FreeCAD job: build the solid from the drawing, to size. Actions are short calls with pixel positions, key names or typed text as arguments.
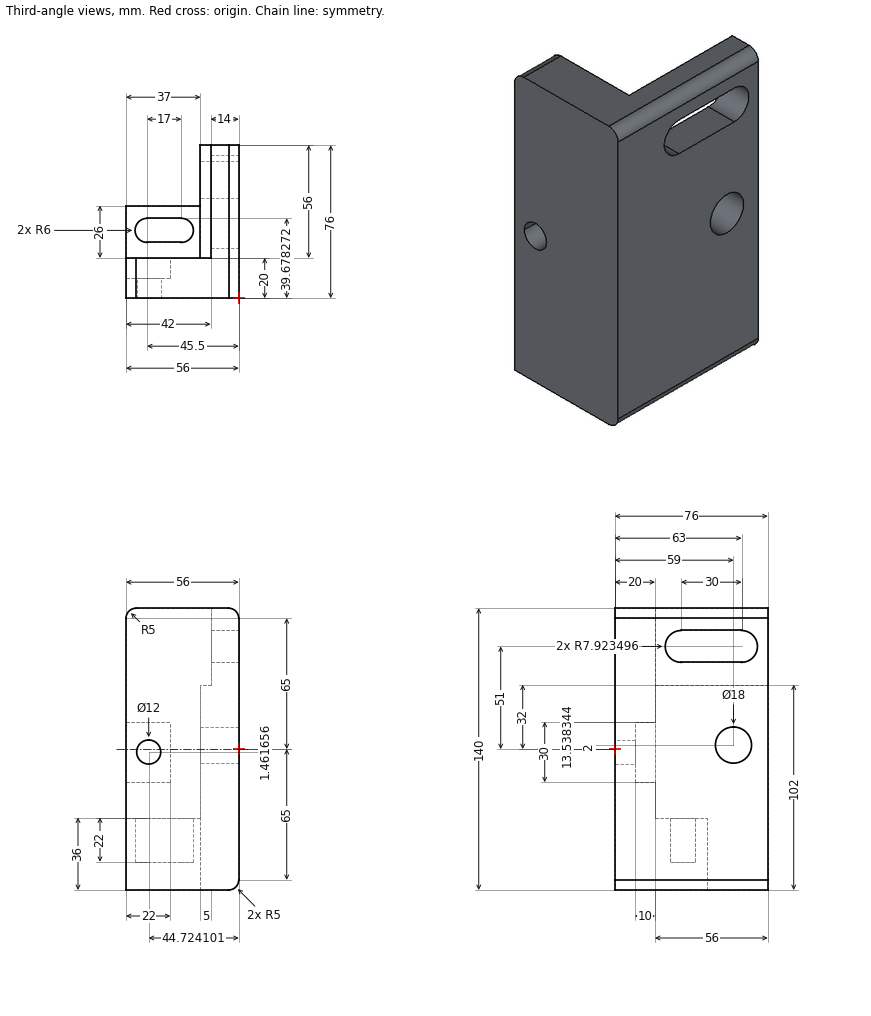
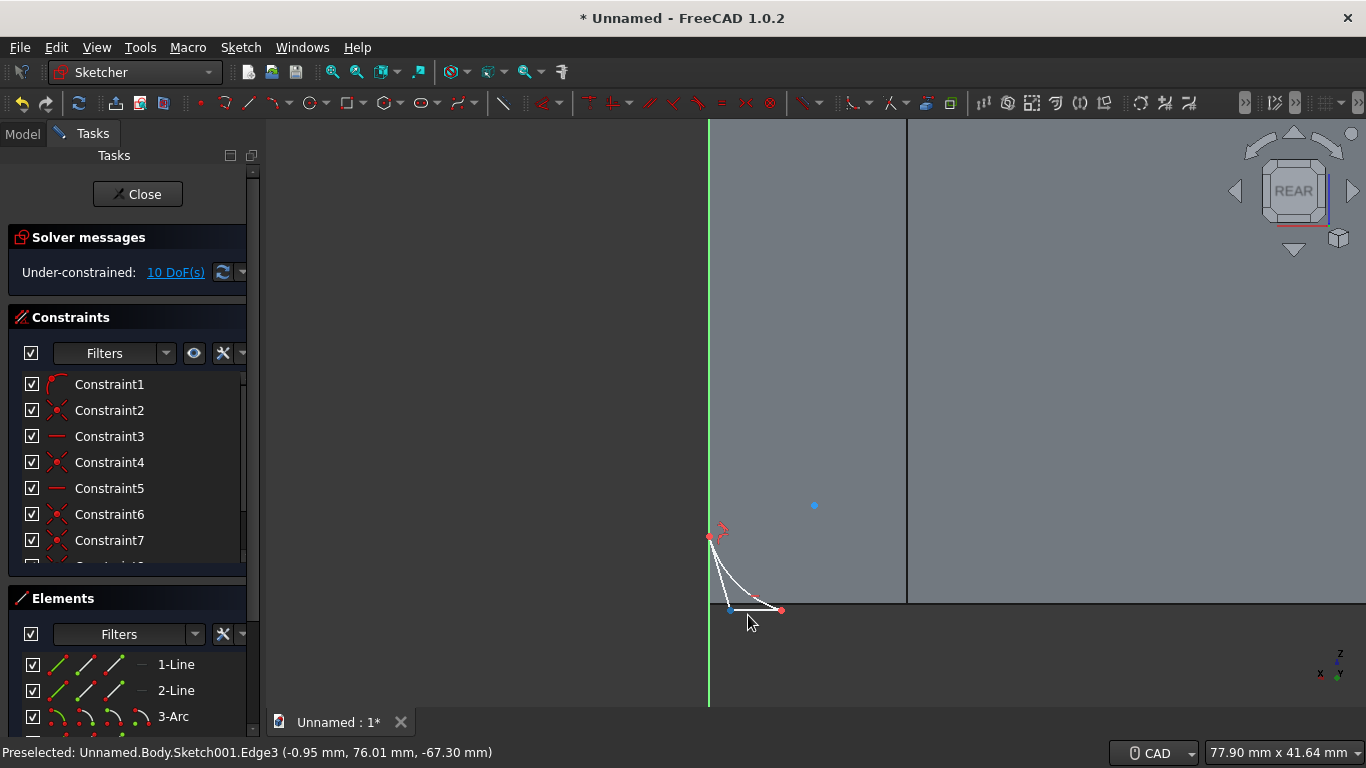
click(746, 610)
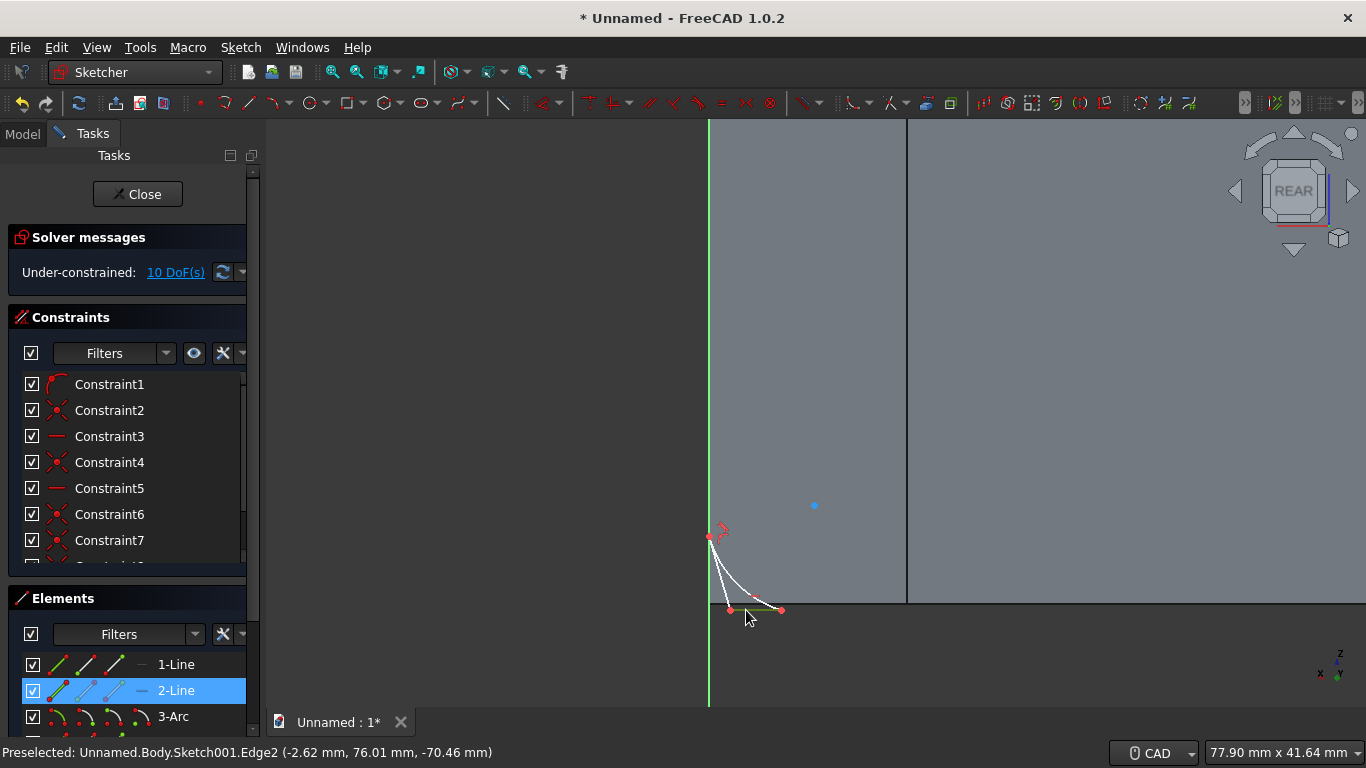
click(736, 582)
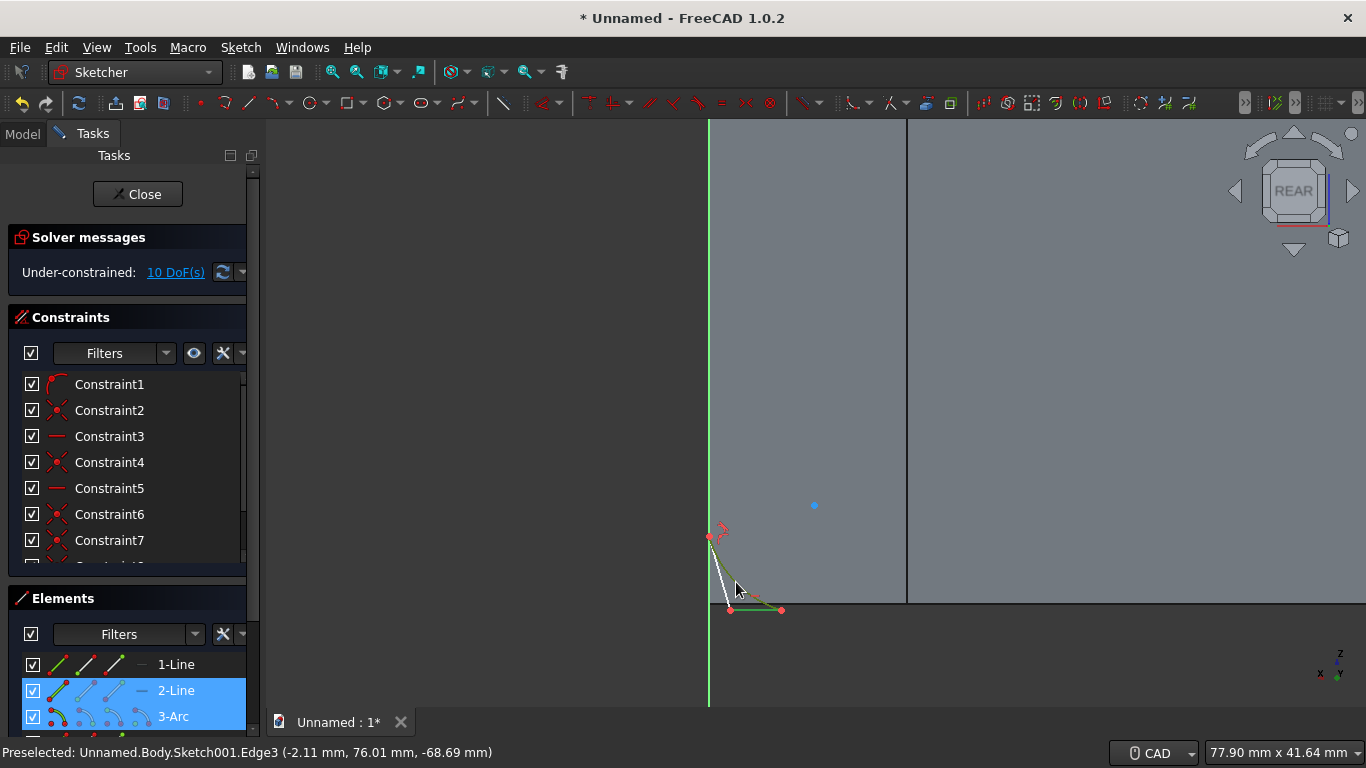
click(698, 104)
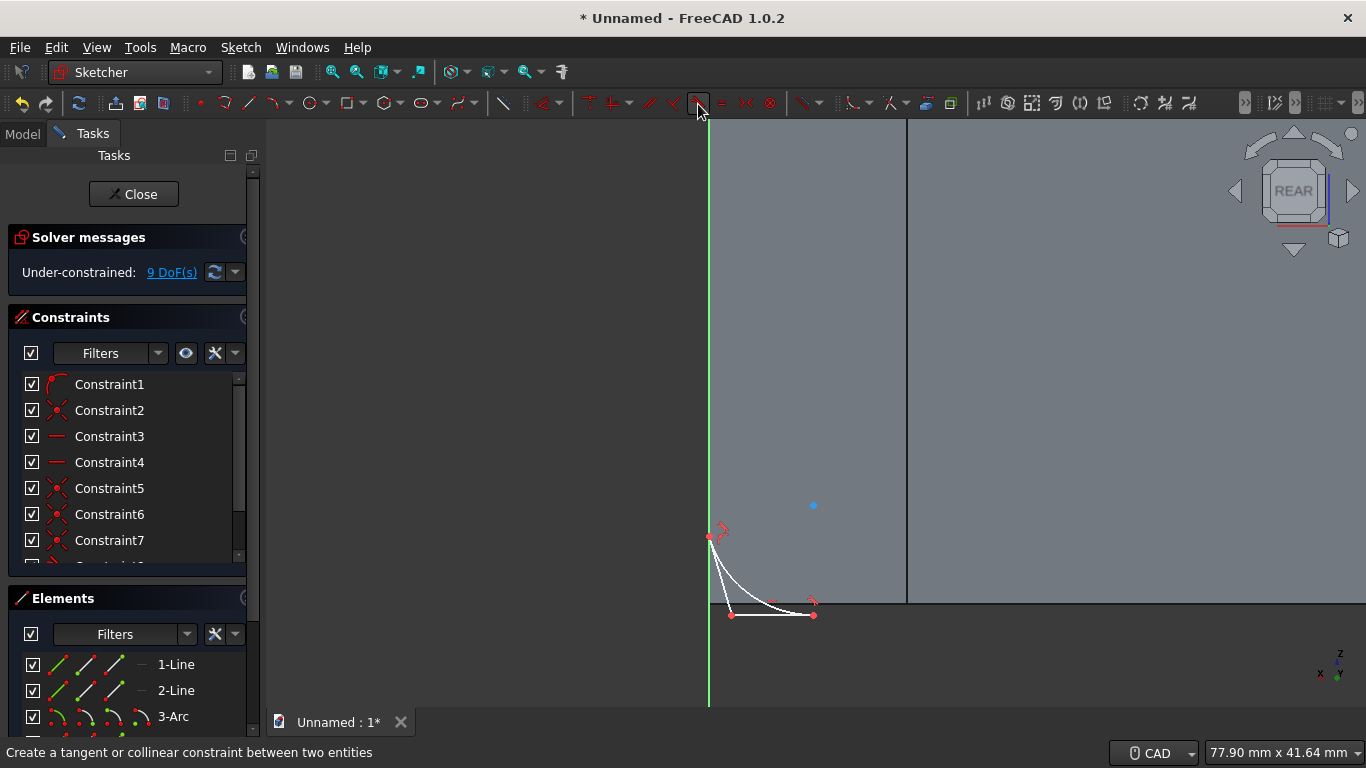
scroll(748, 615, down, 8)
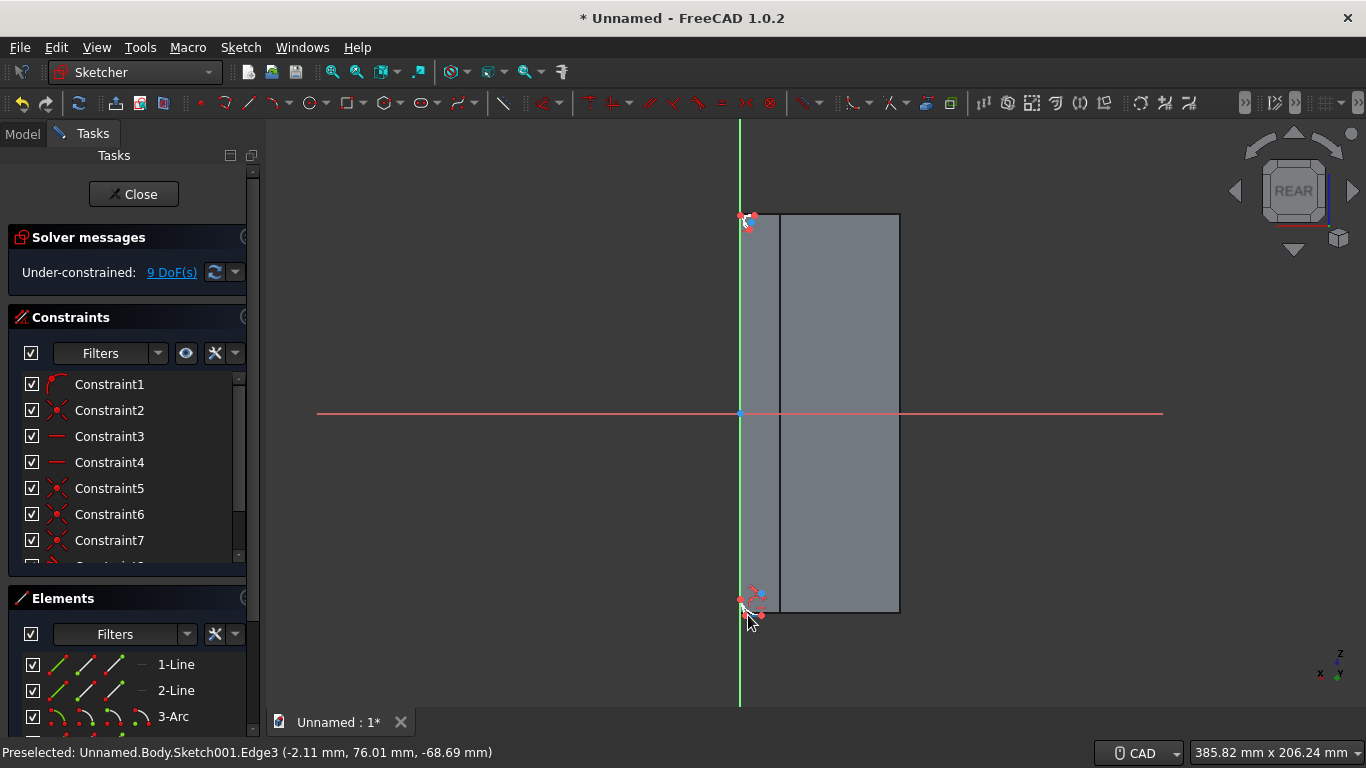
scroll(743, 216, up, 9)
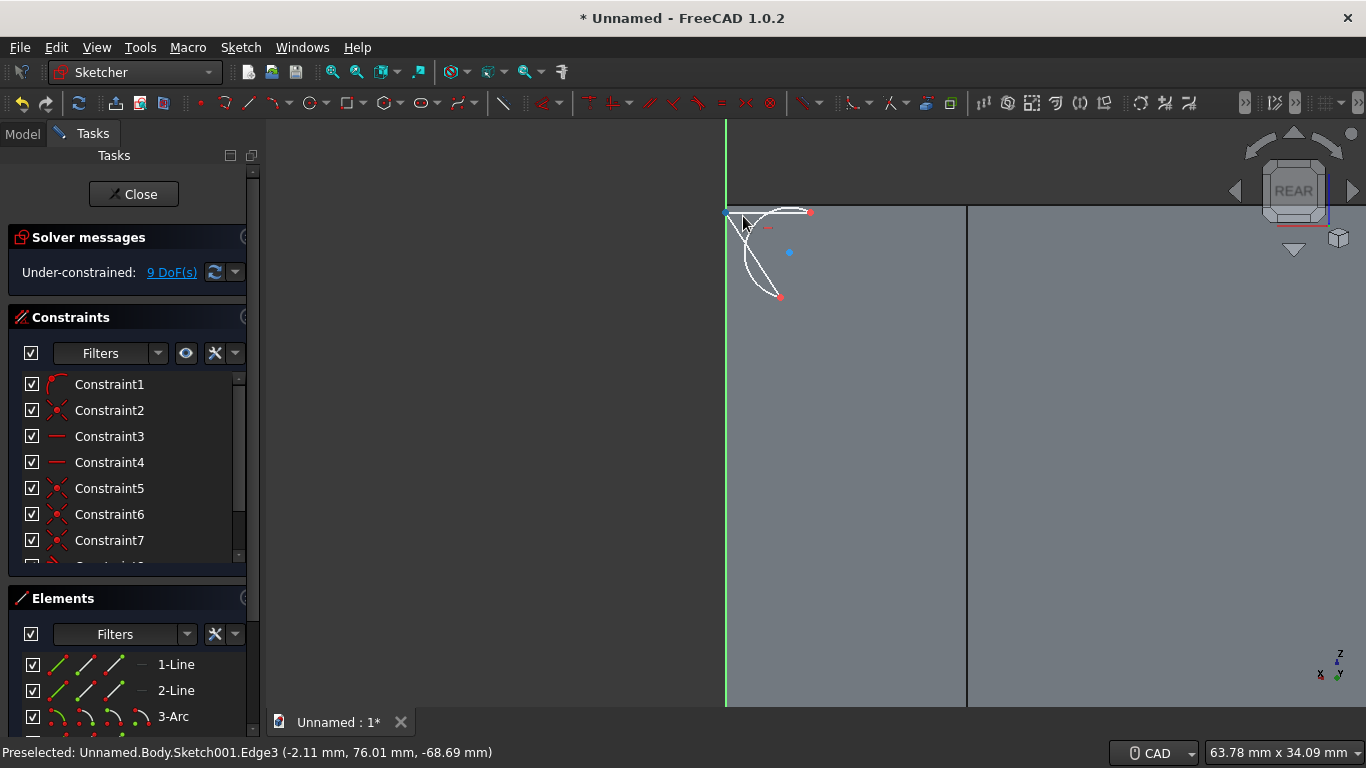
click(743, 213)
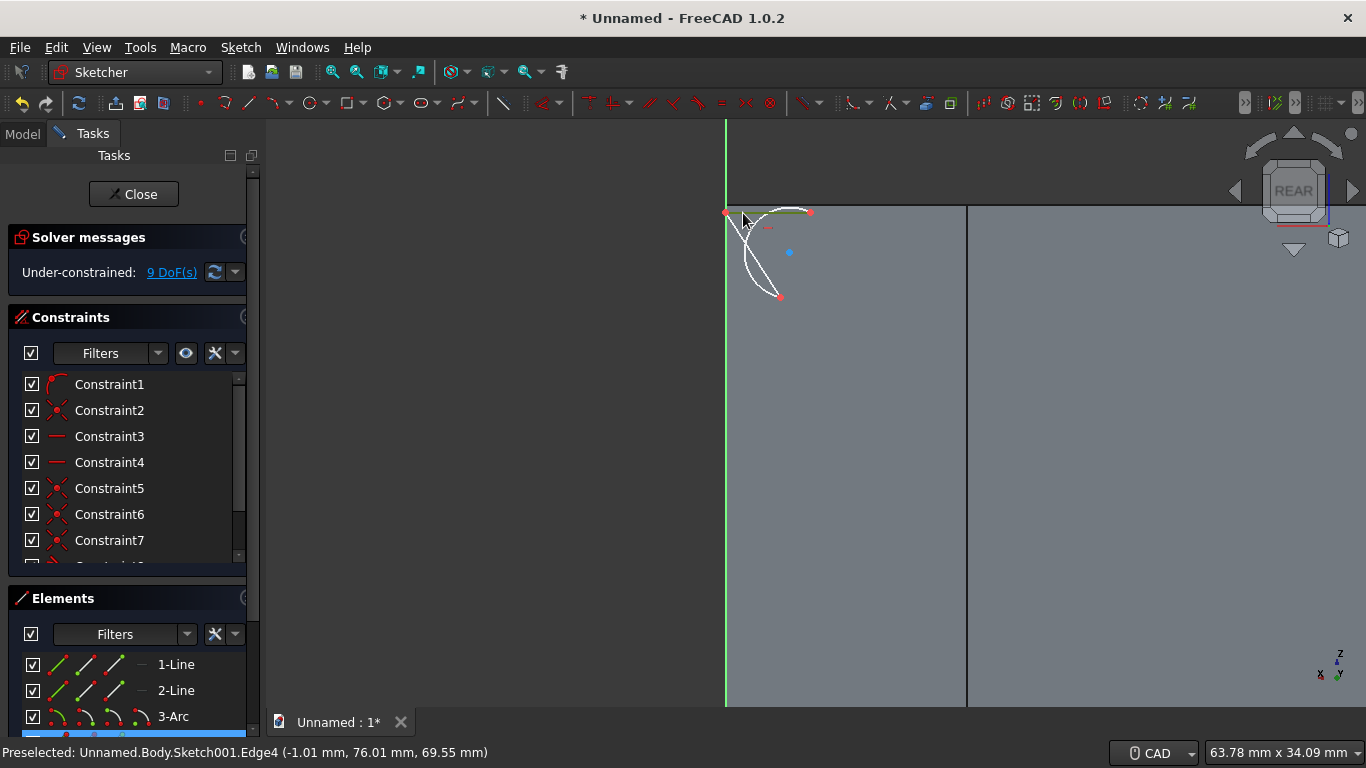
click(747, 268)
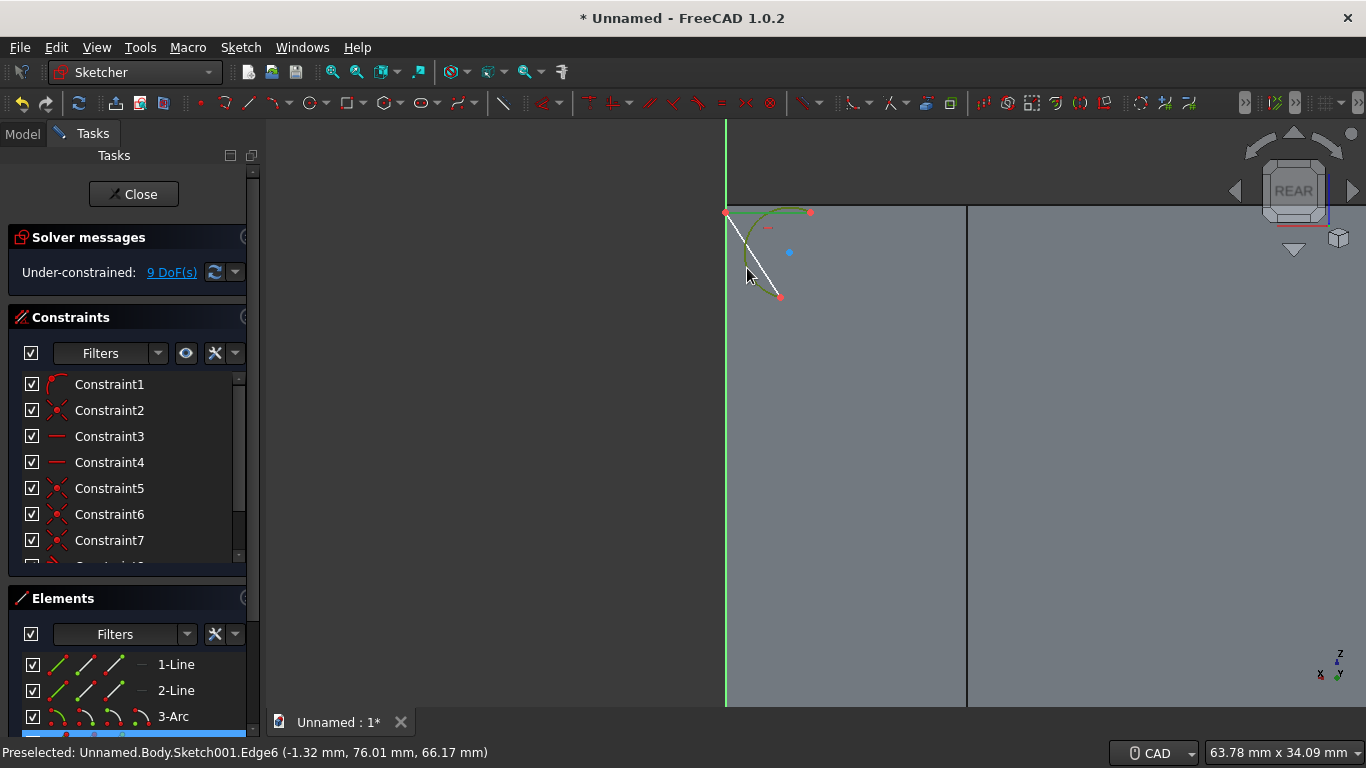
click(698, 104)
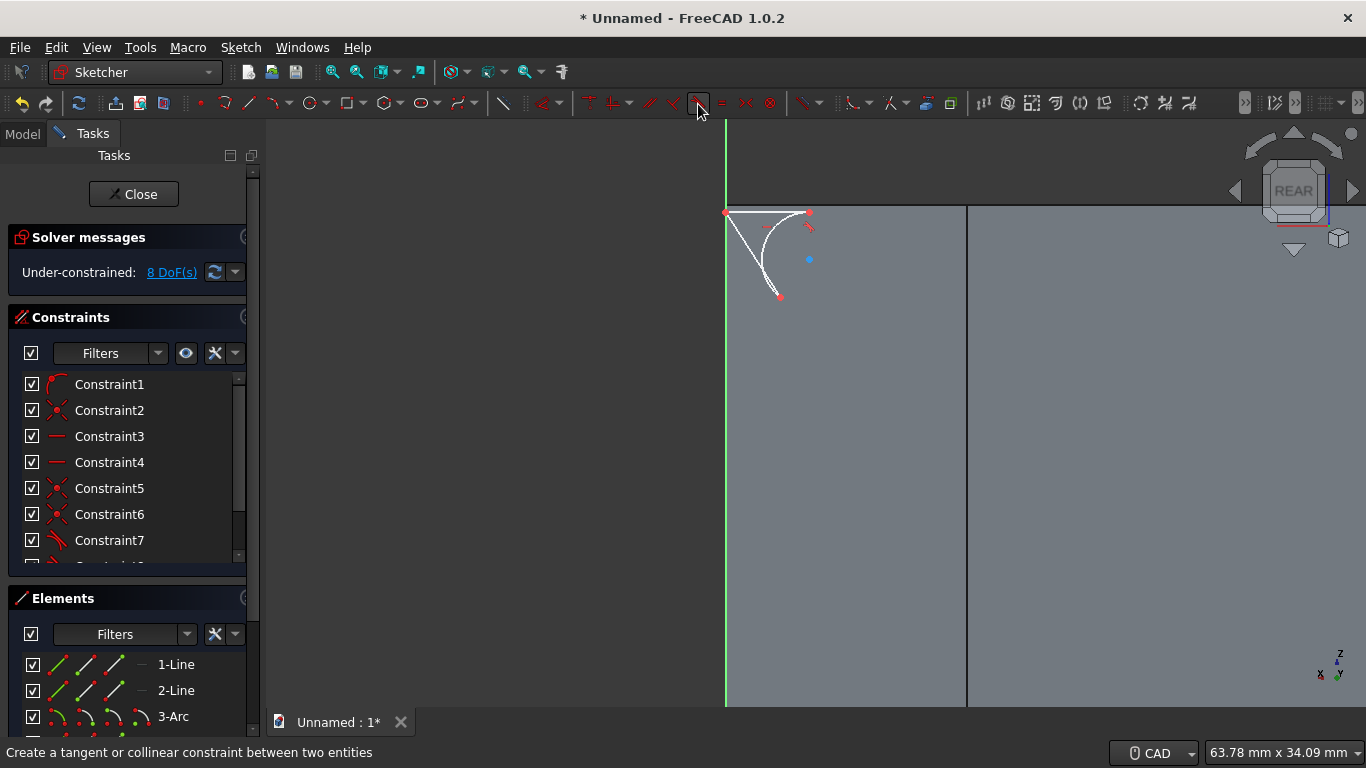
click(742, 238)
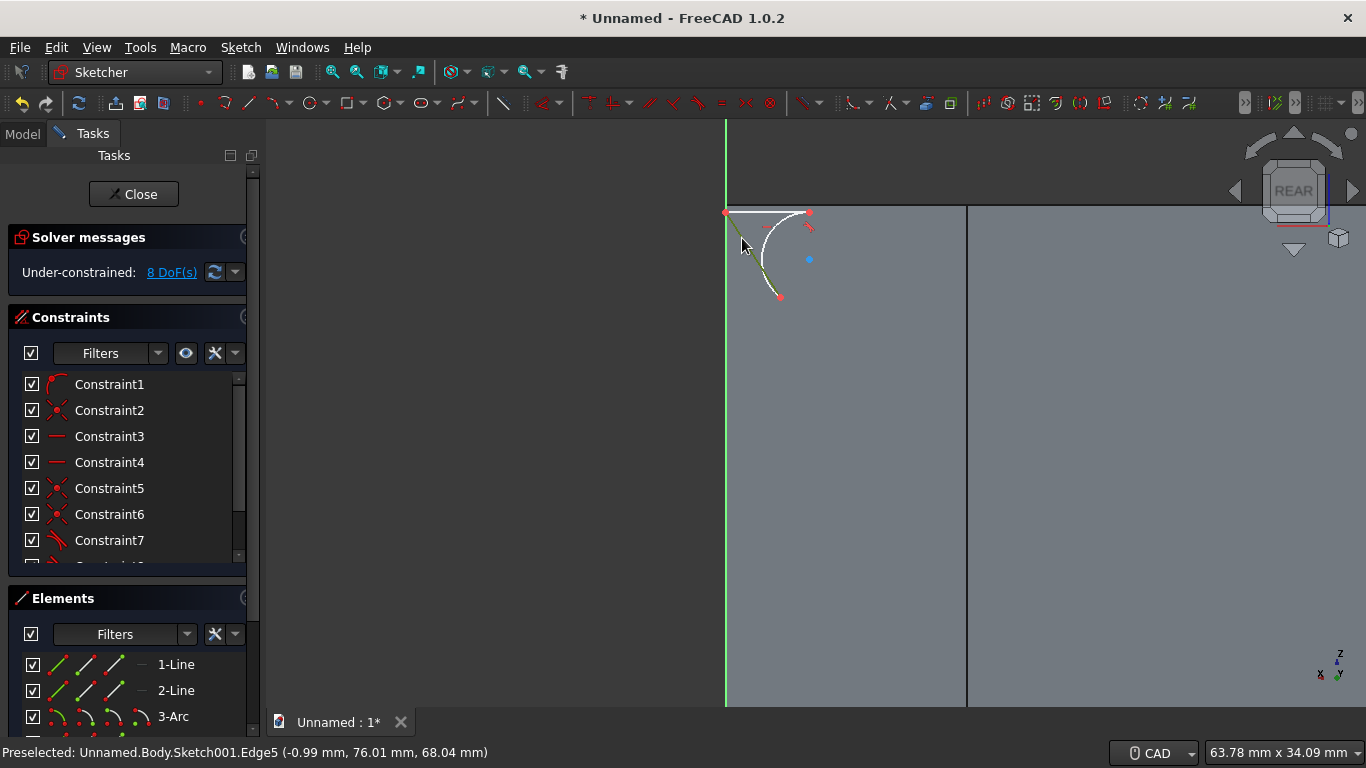
click(777, 225)